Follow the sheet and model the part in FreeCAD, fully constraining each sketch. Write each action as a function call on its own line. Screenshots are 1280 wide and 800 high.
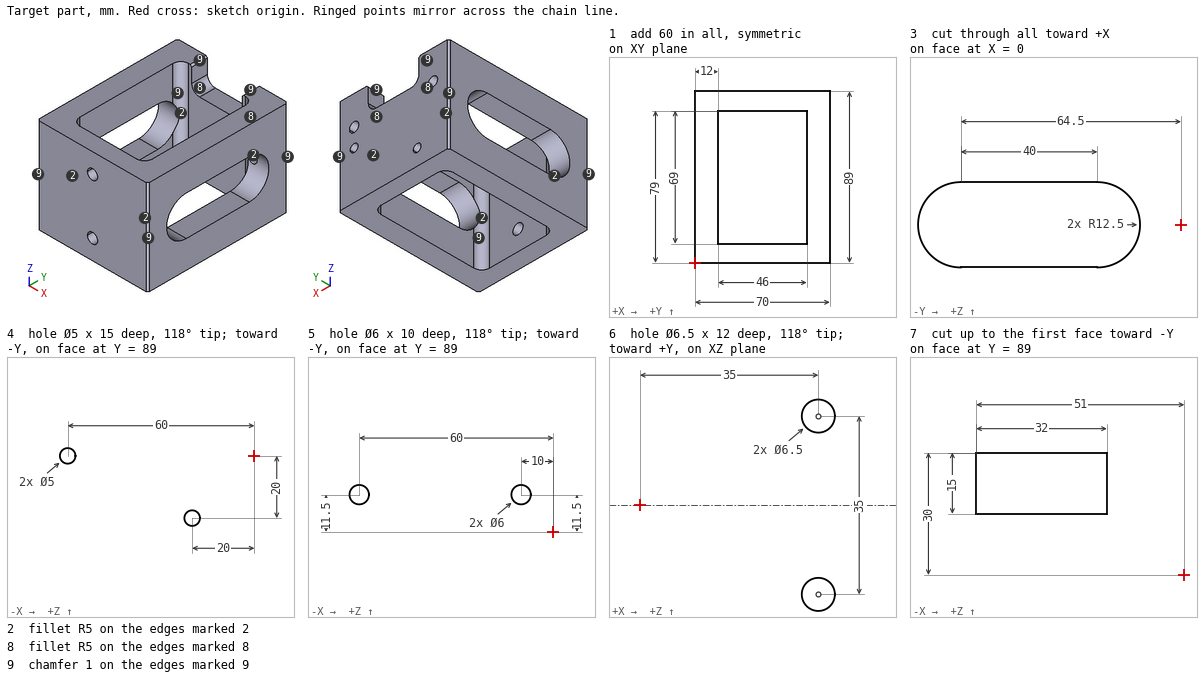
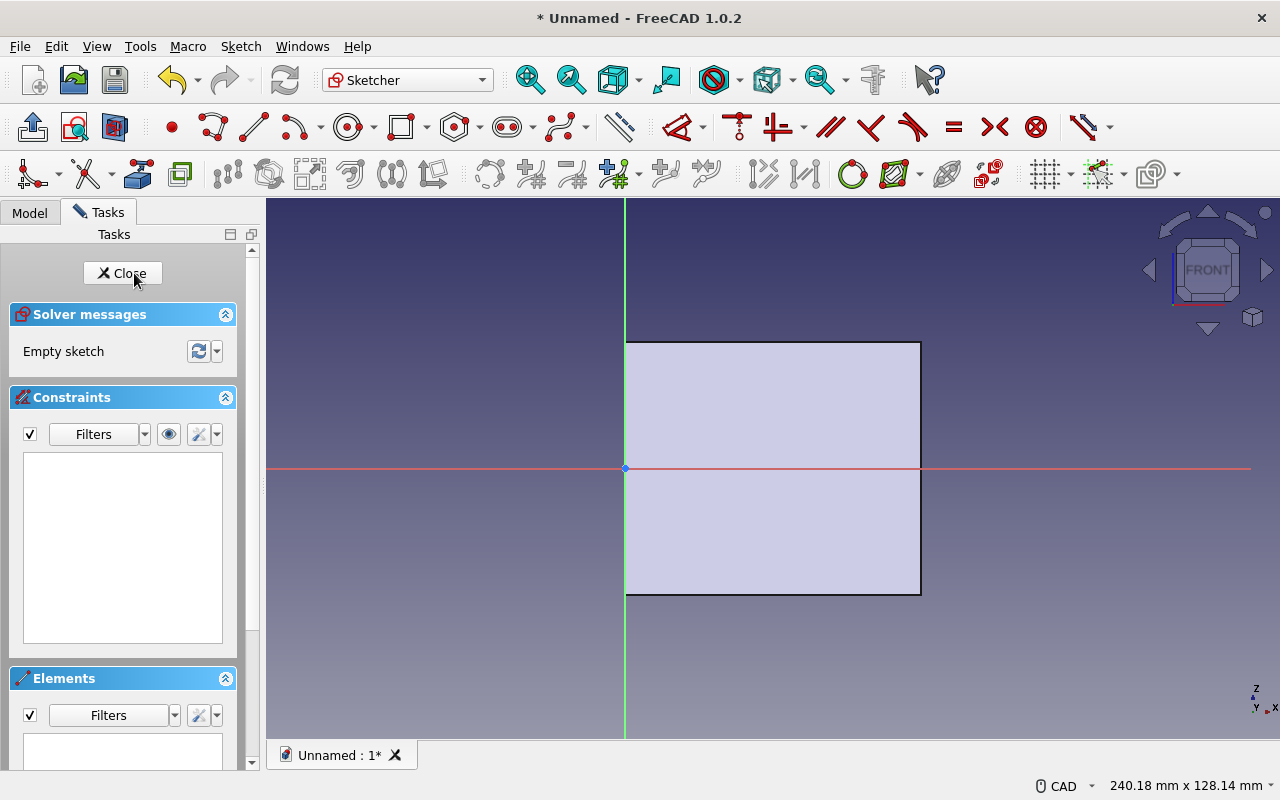
scroll(708, 469, up, 3)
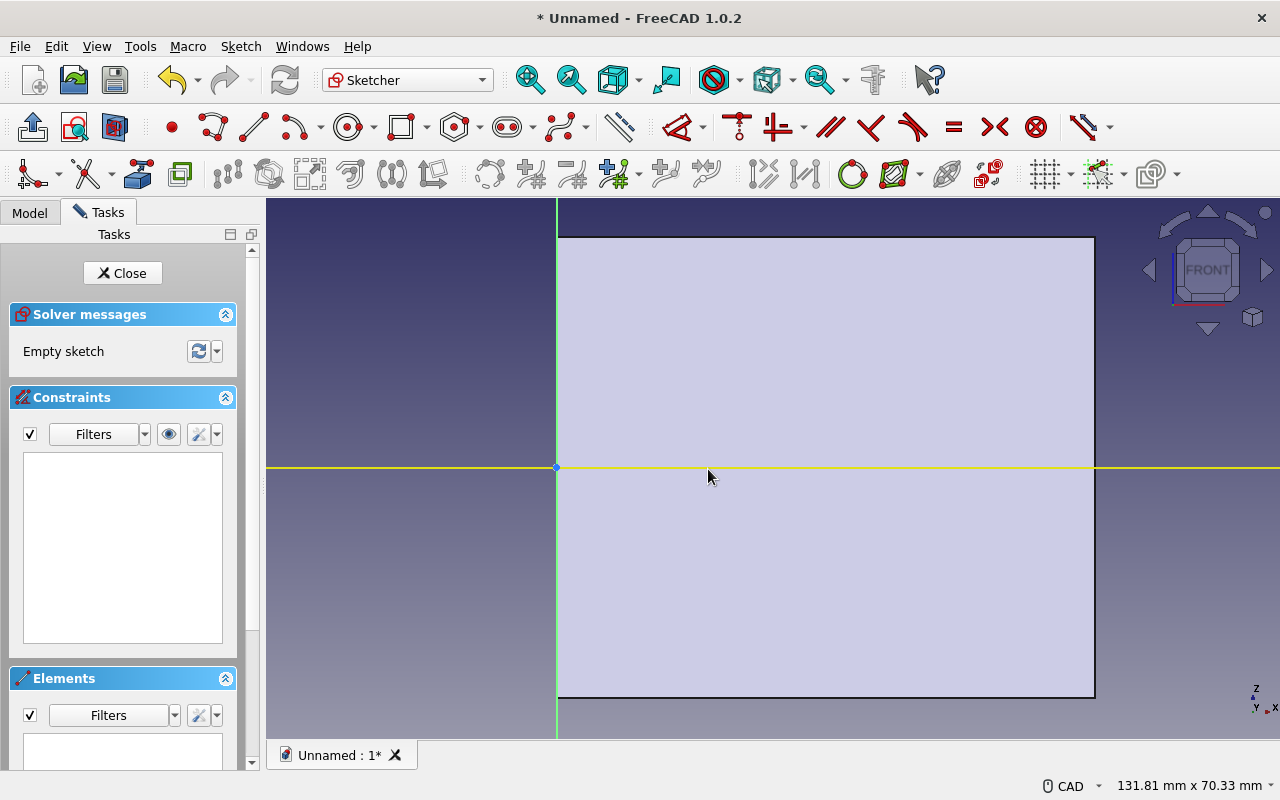
click(348, 128)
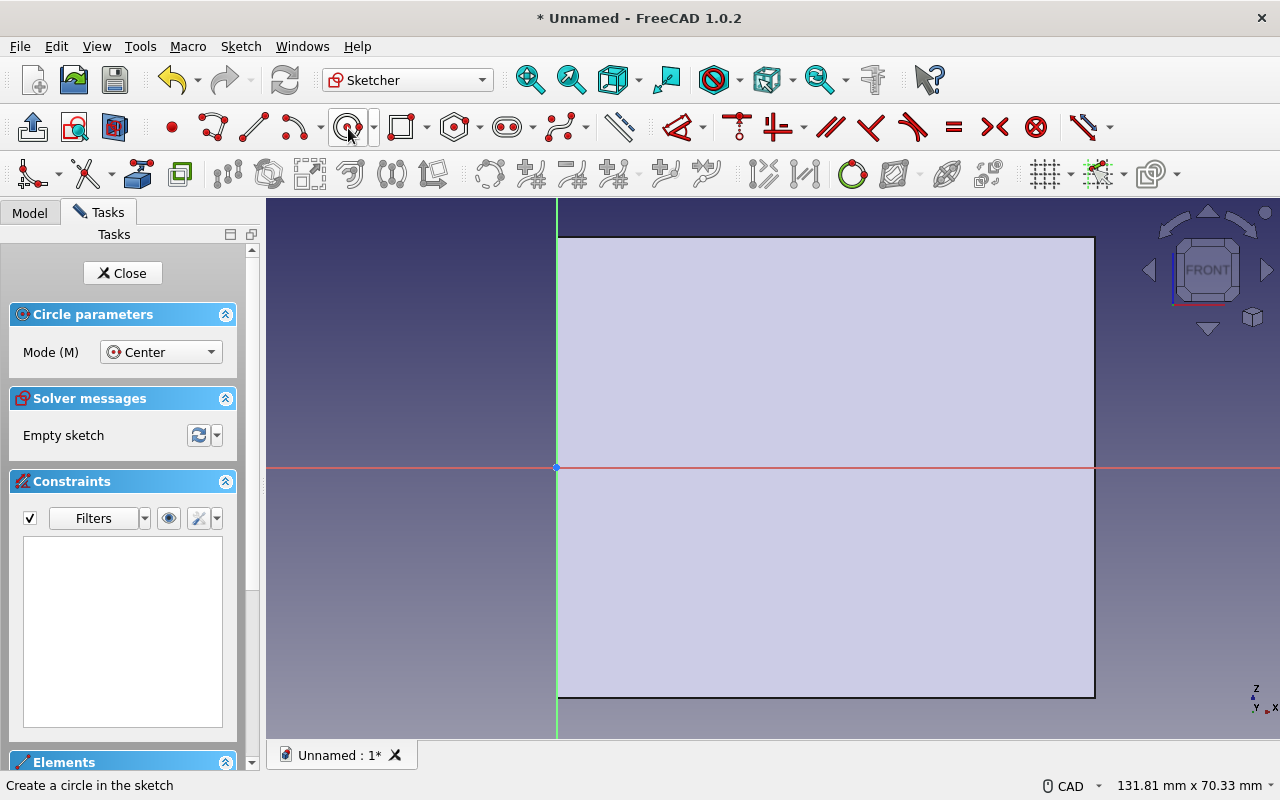
click(826, 333)
click(844, 315)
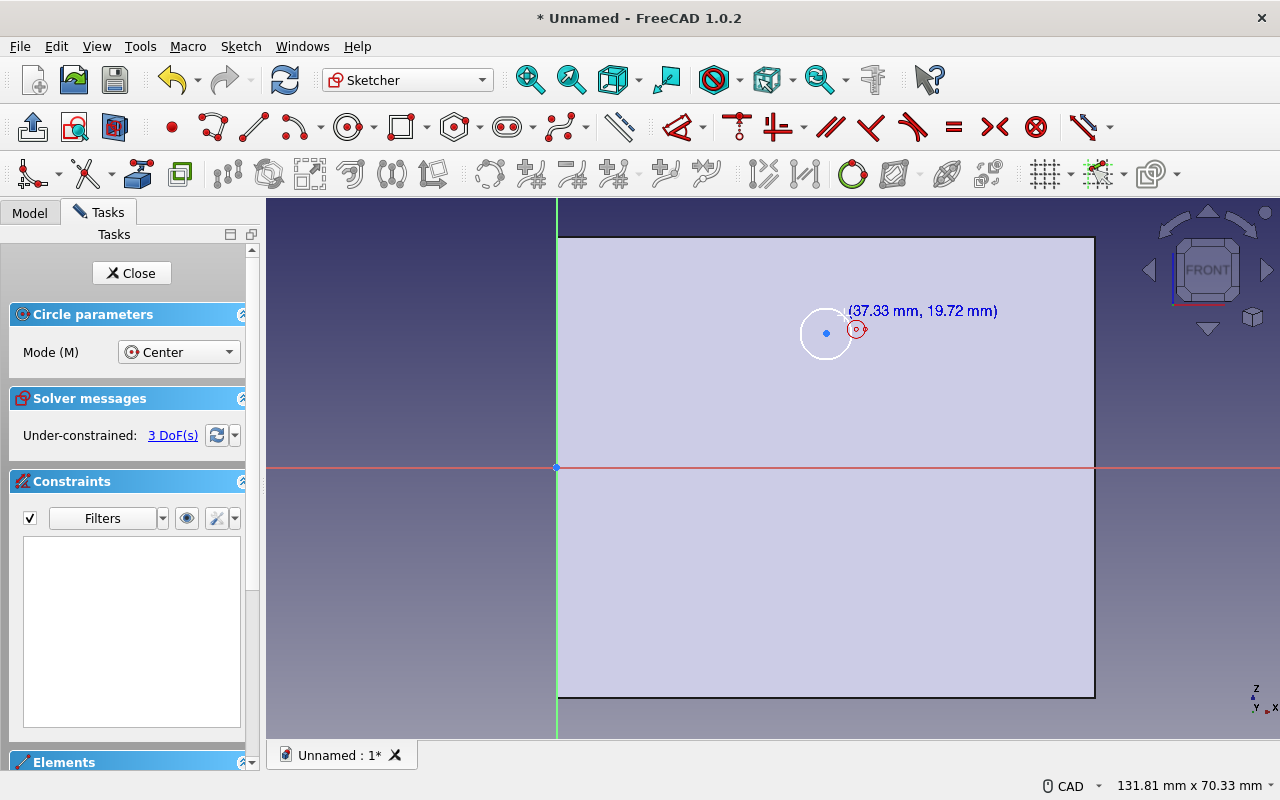
click(826, 602)
click(844, 585)
key(Escape)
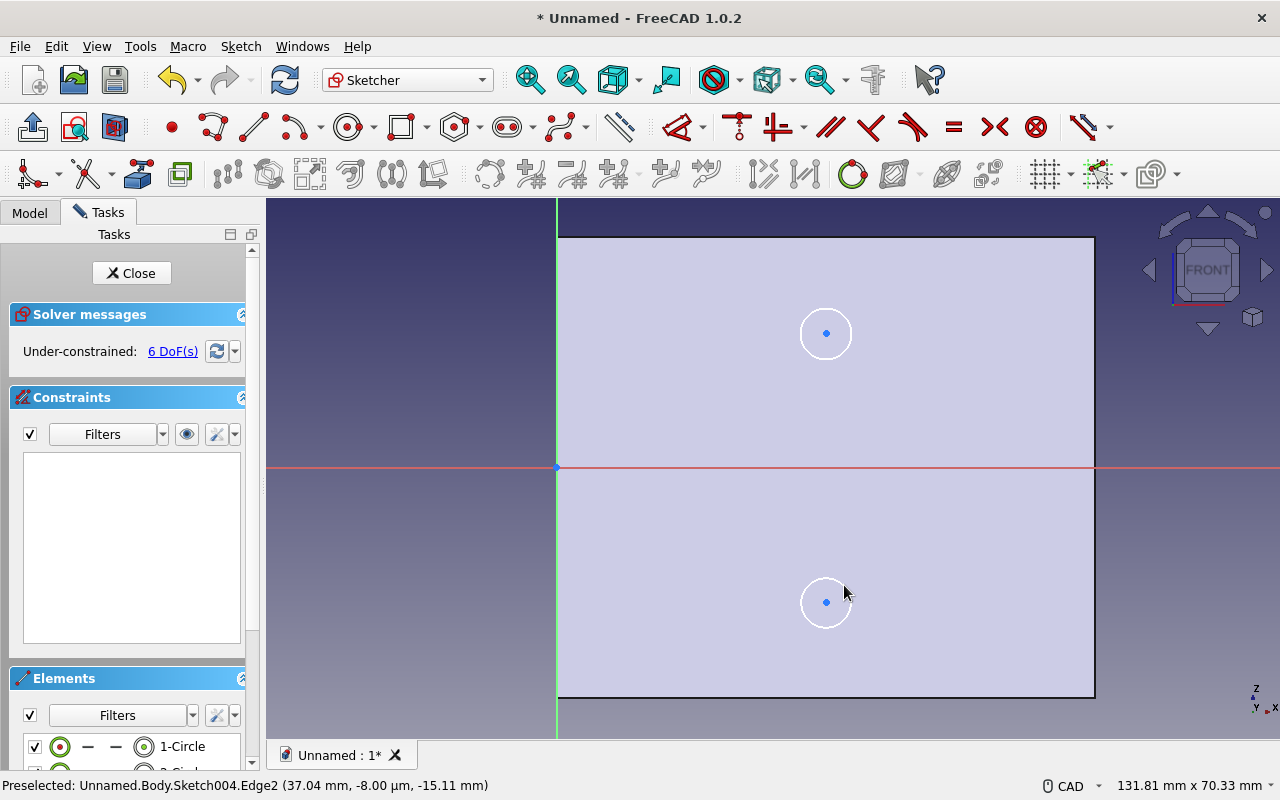
click(844, 316)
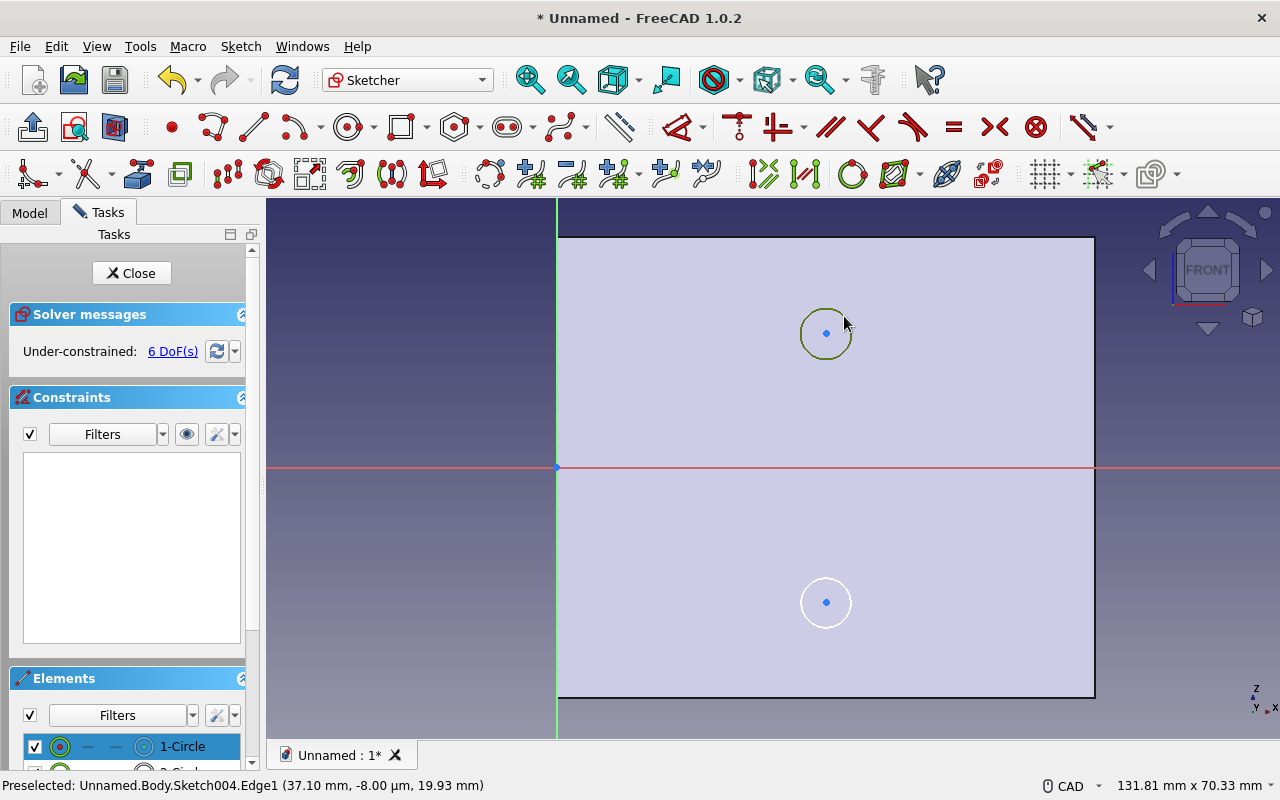
click(843, 585)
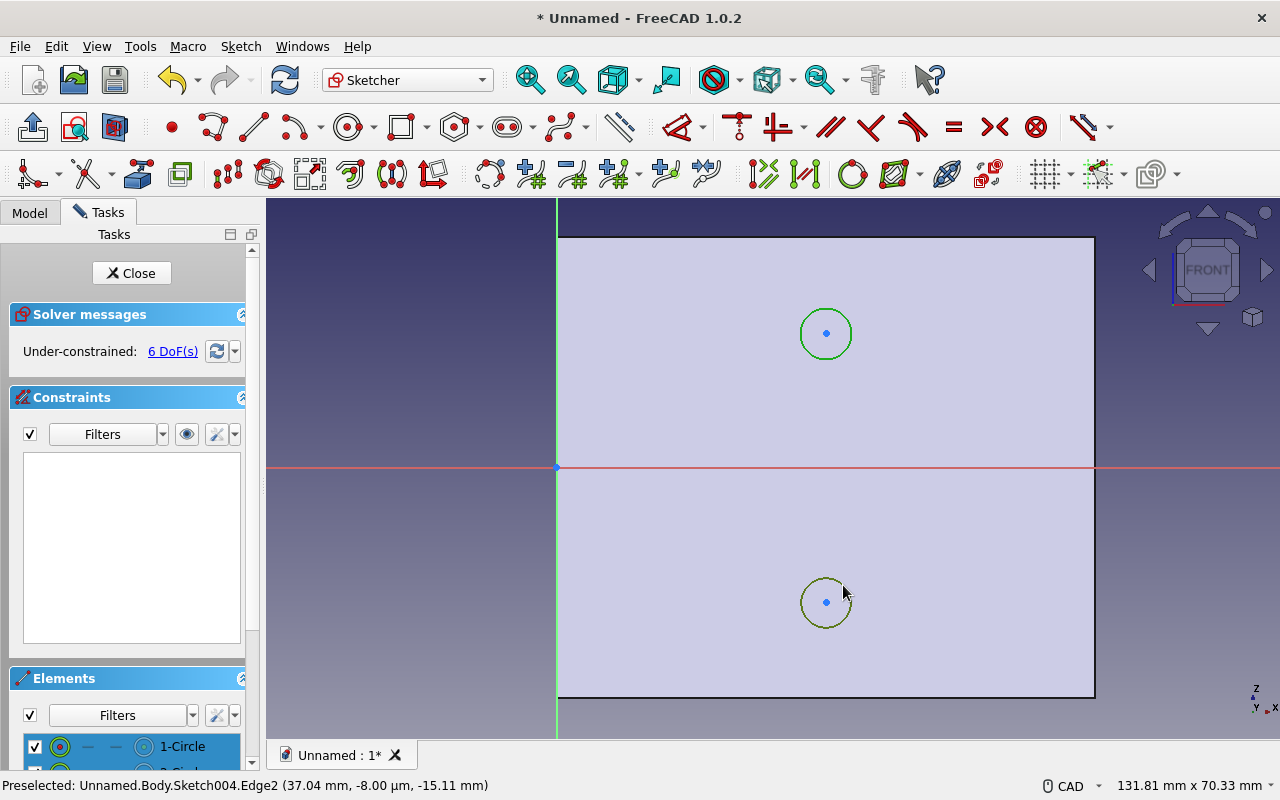
key(e)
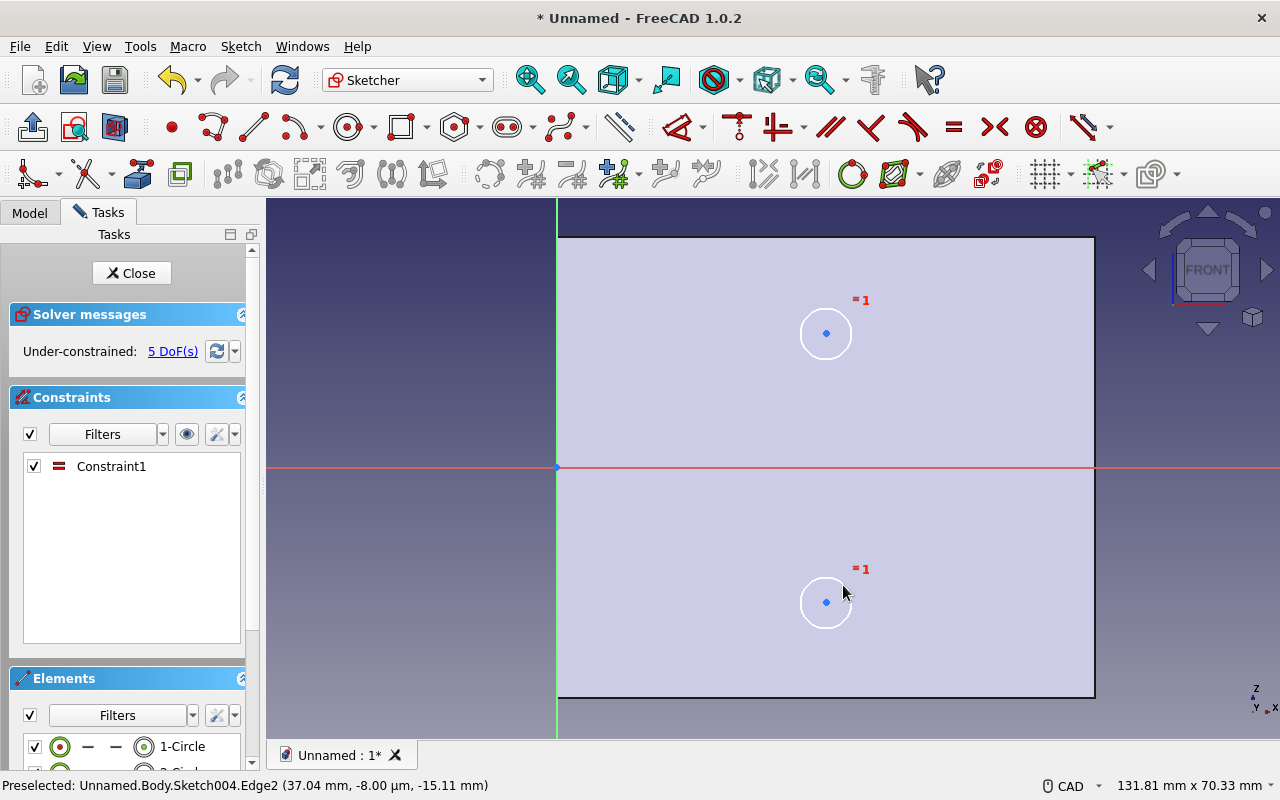
click(826, 334)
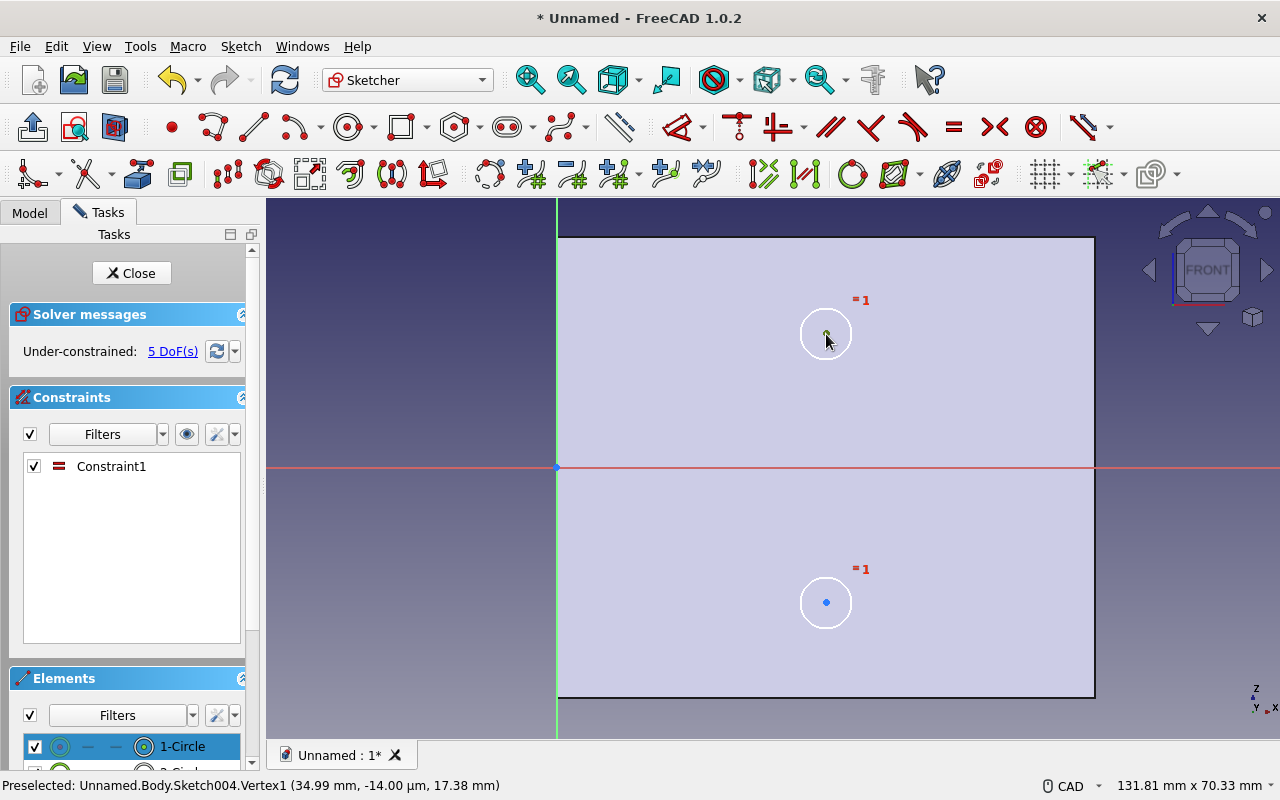
click(826, 603)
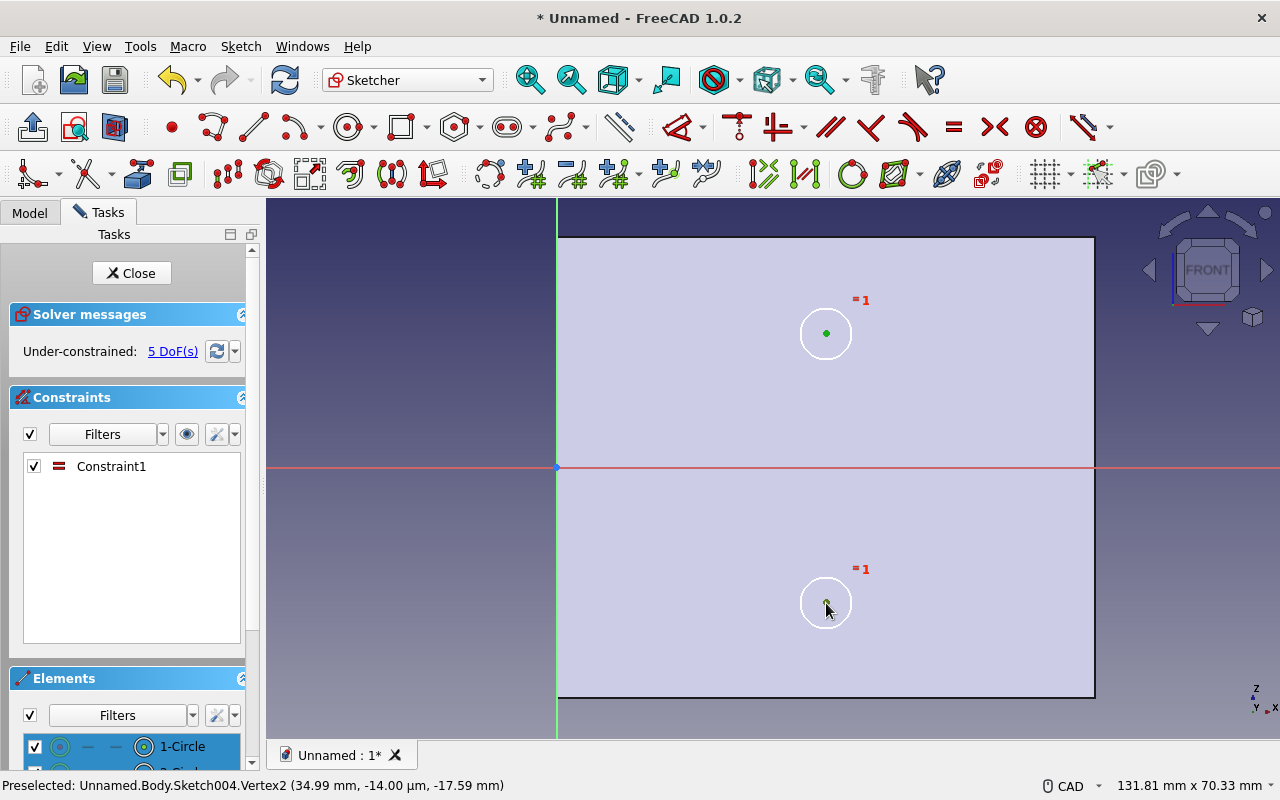
click(353, 468)